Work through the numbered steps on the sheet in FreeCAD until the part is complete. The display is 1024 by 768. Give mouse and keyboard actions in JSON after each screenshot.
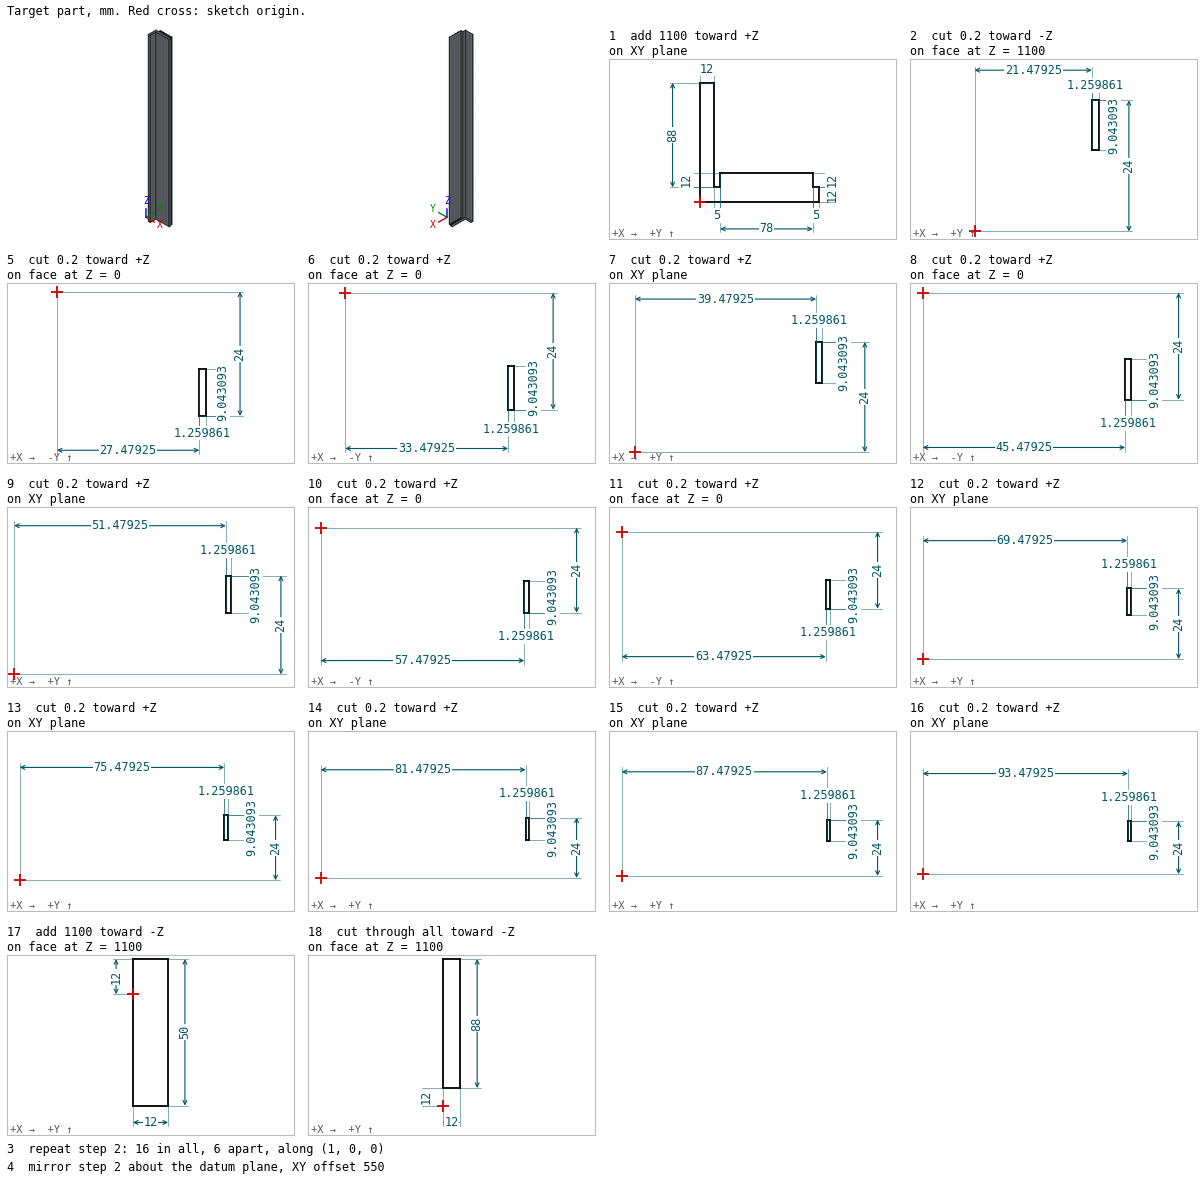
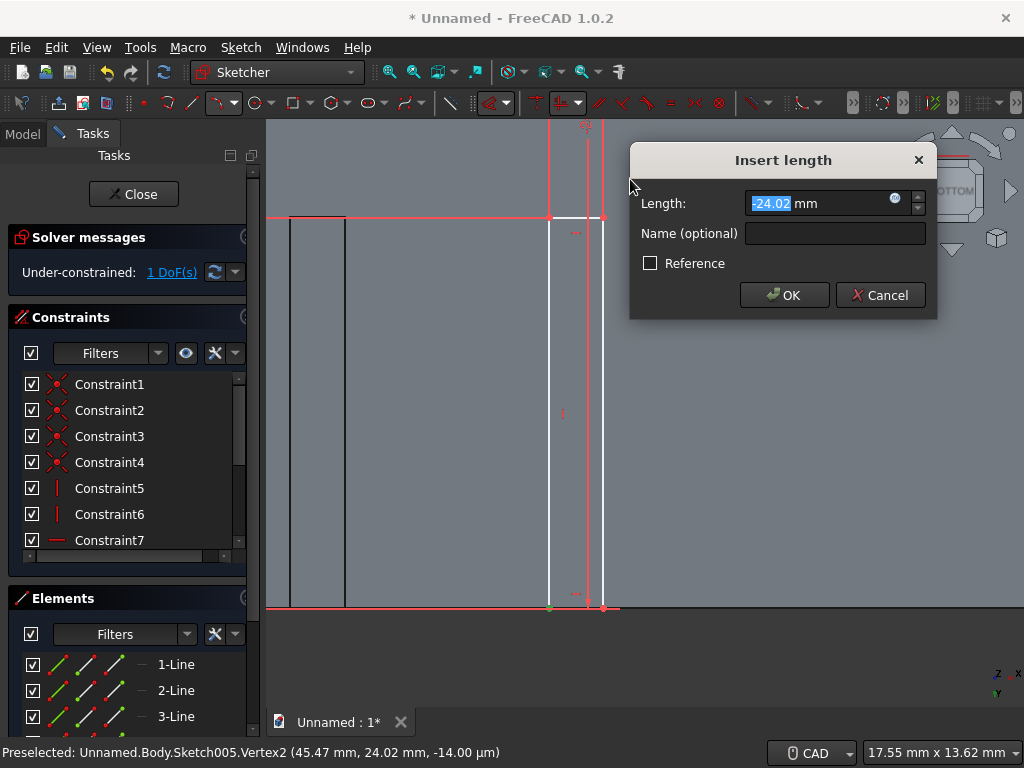
{"action": "type", "text": "-24"}
{"action": "key", "text": "Return"}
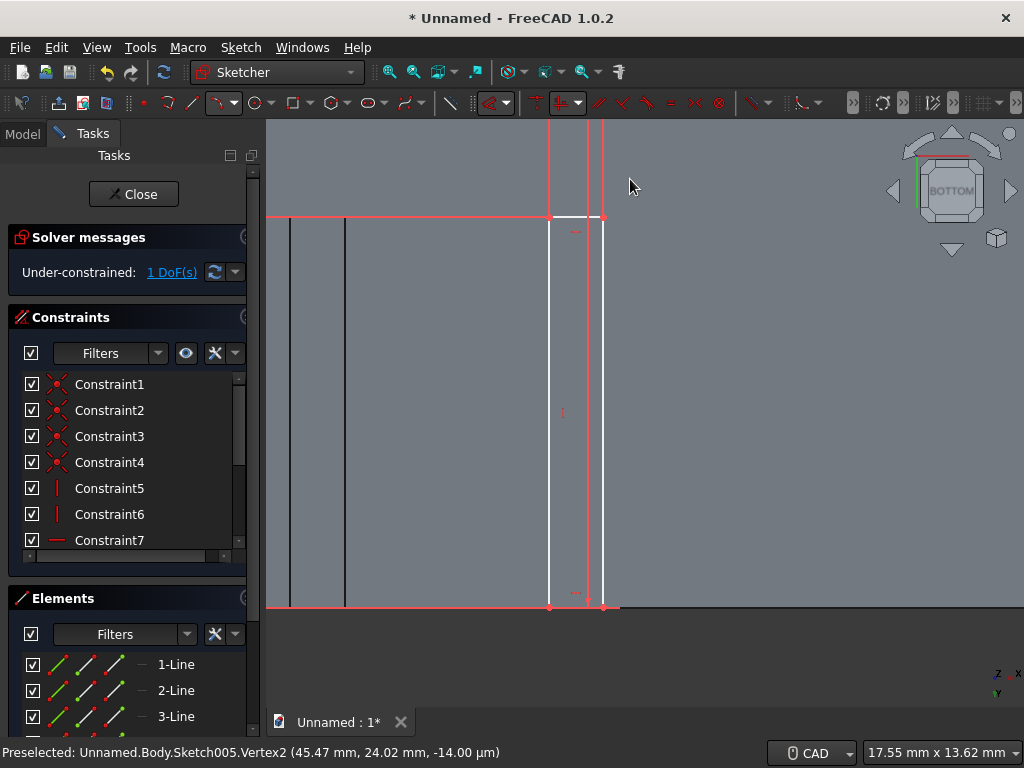
{"action": "left_click", "coordinate": [549, 217]}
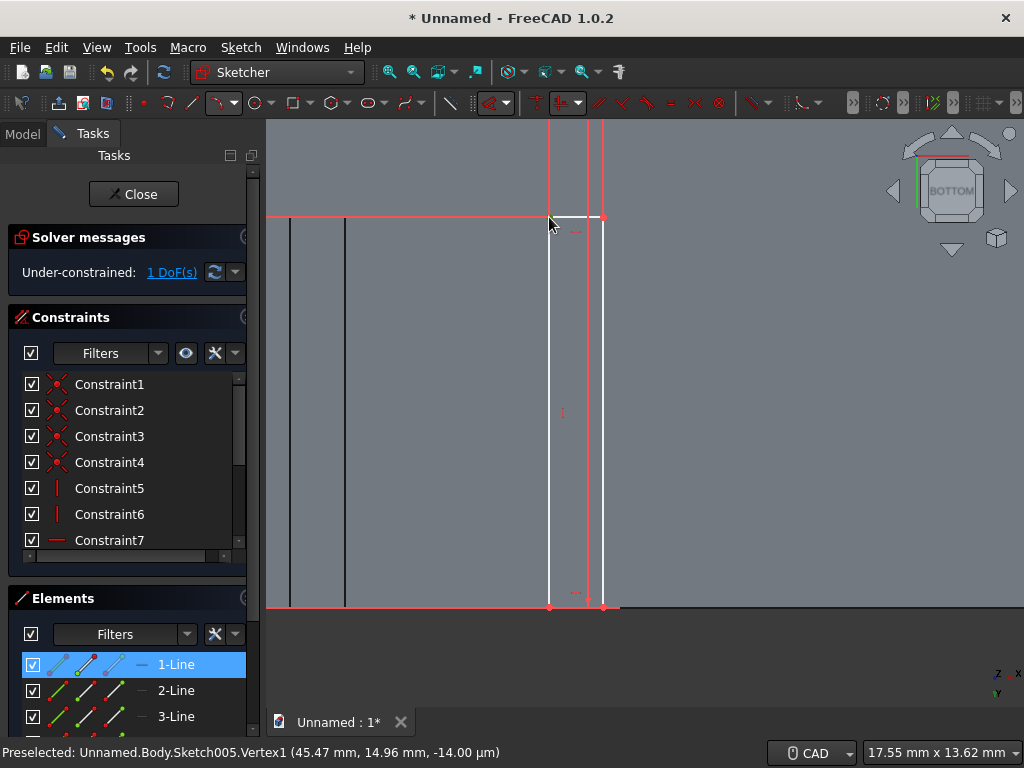
{"action": "left_click", "coordinate": [508, 104]}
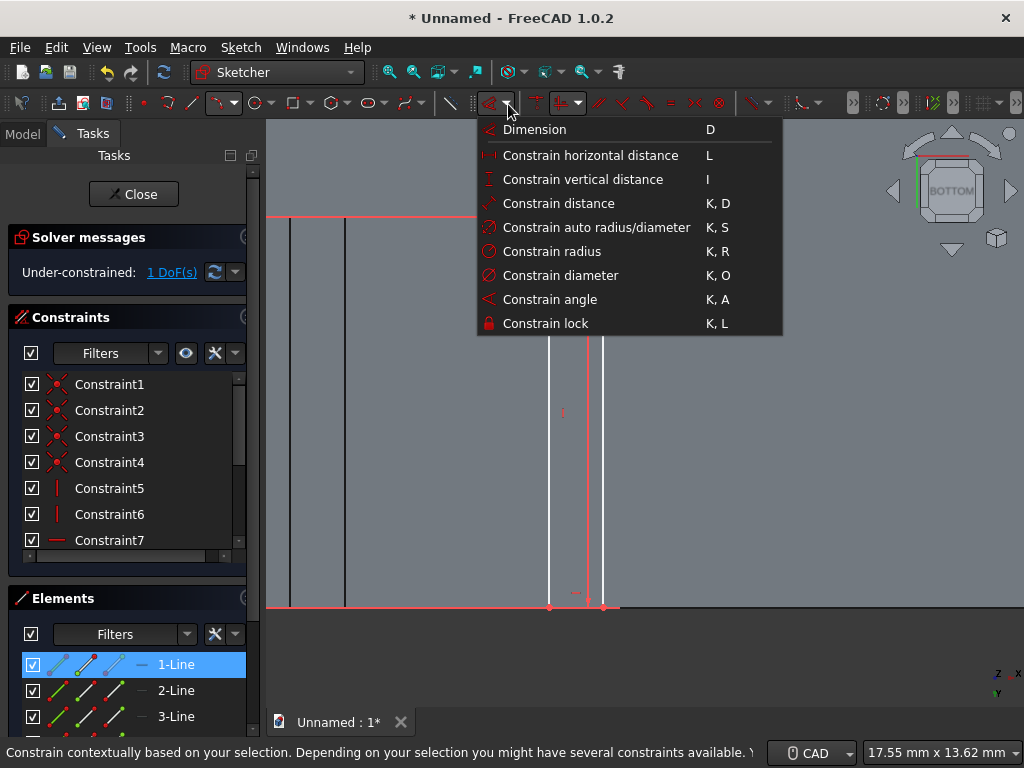
{"action": "left_click", "coordinate": [630, 155]}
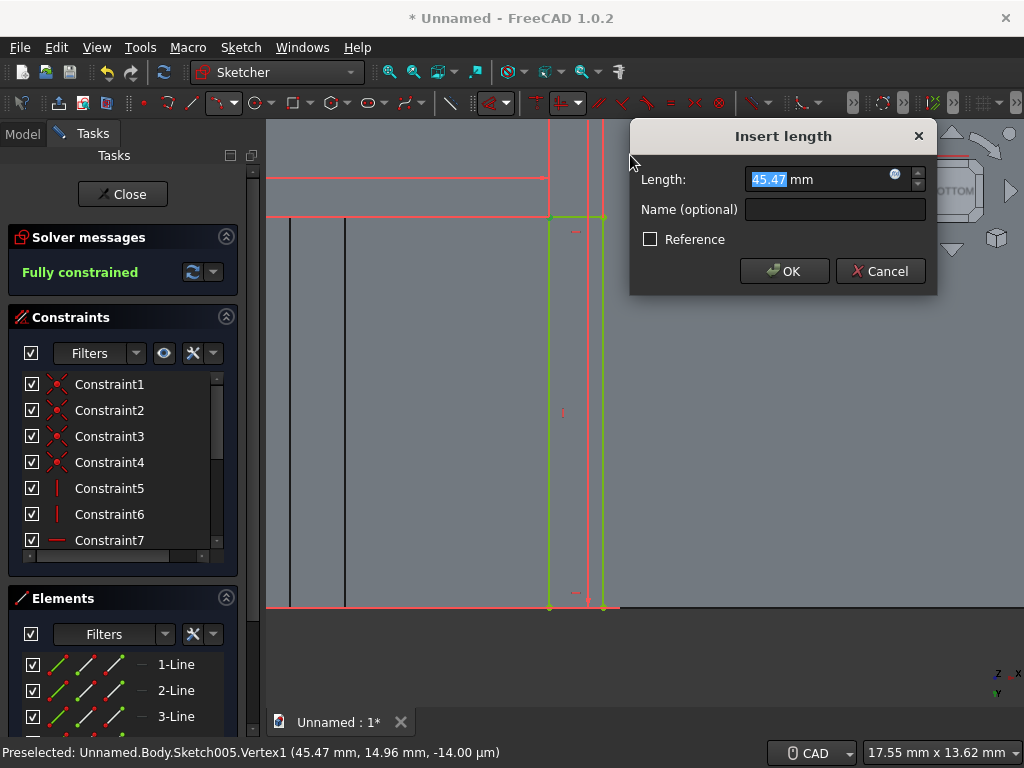
{"action": "type", "text": "45.47925"}
{"action": "key", "text": "Return"}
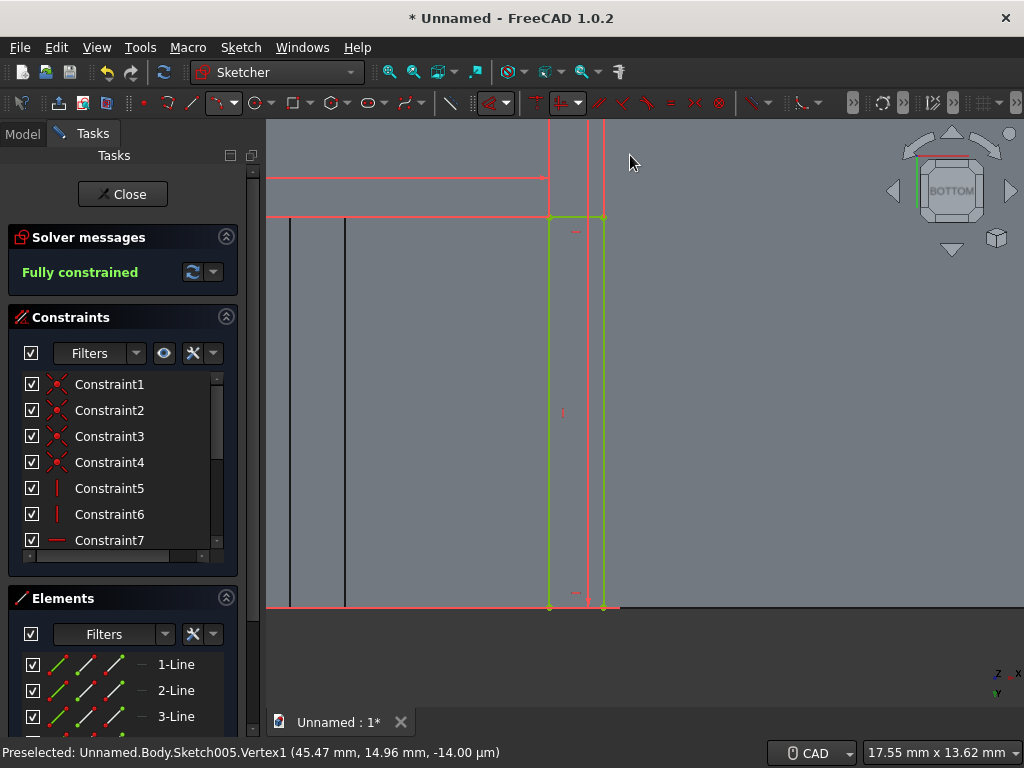
{"action": "left_click", "coordinate": [123, 194]}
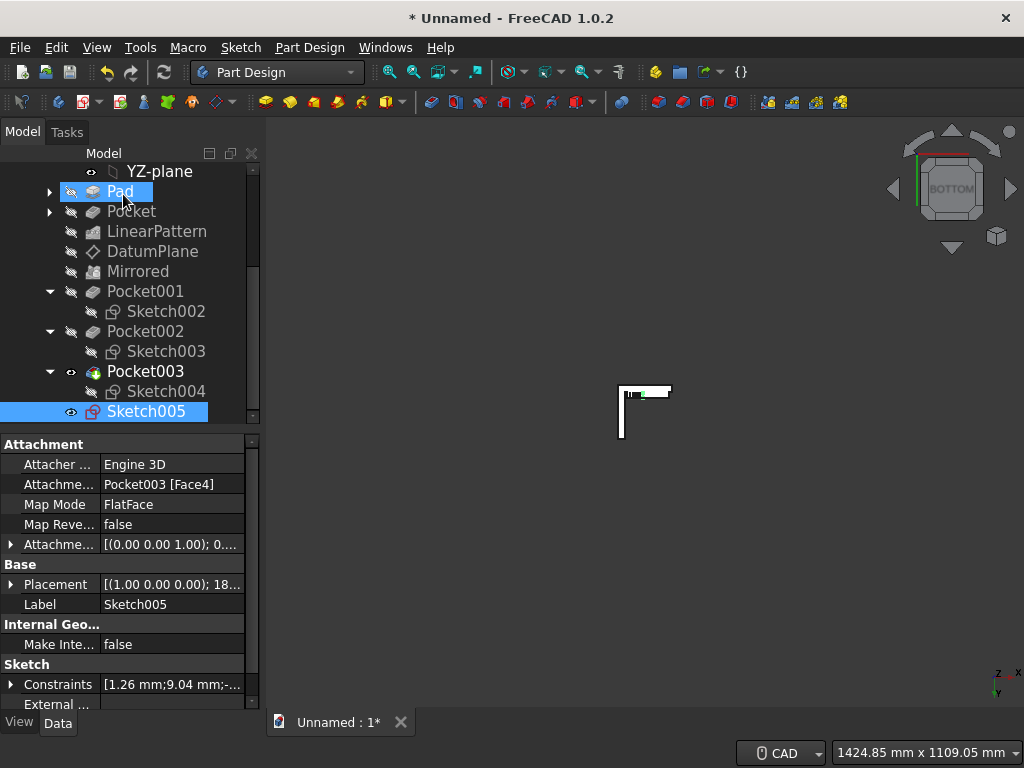
{"action": "left_click", "coordinate": [432, 102]}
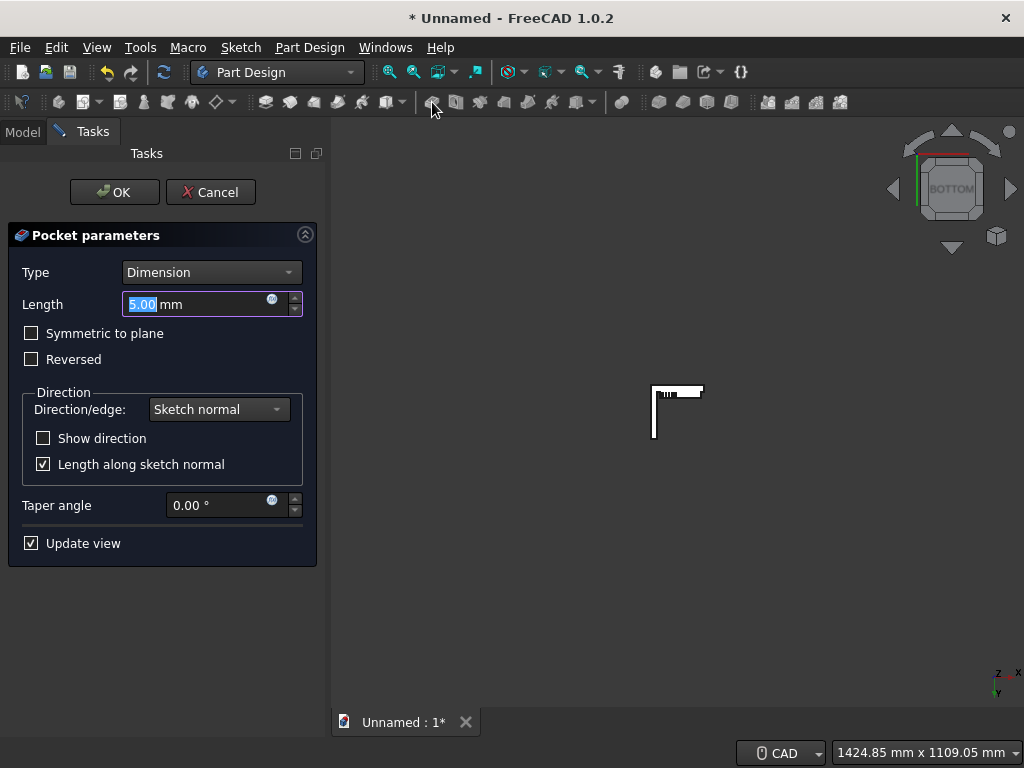
{"action": "type", "text": "0.2"}
{"action": "key", "text": "Tab"}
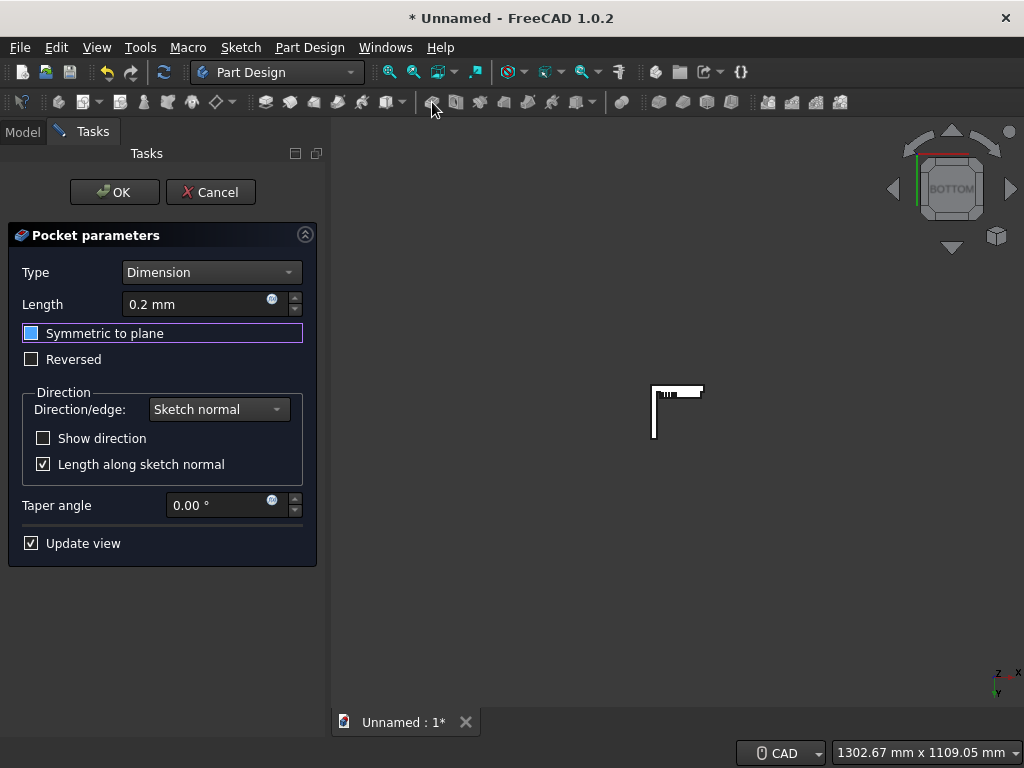
{"action": "left_click", "coordinate": [115, 192]}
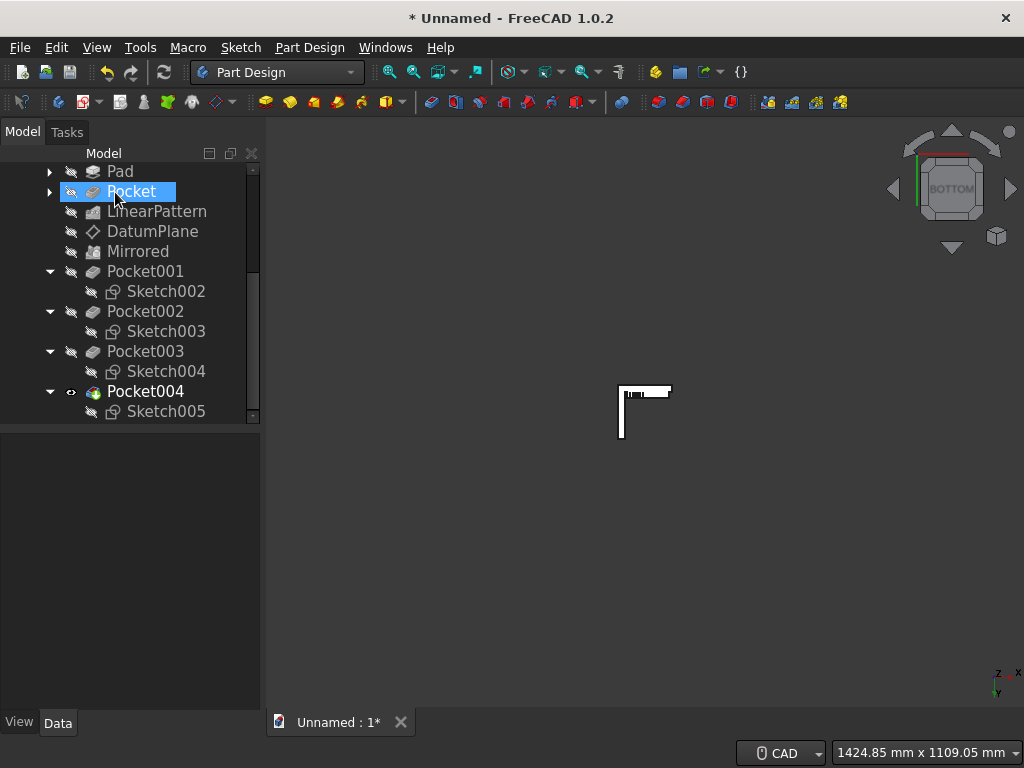
{"action": "left_click", "coordinate": [390, 72]}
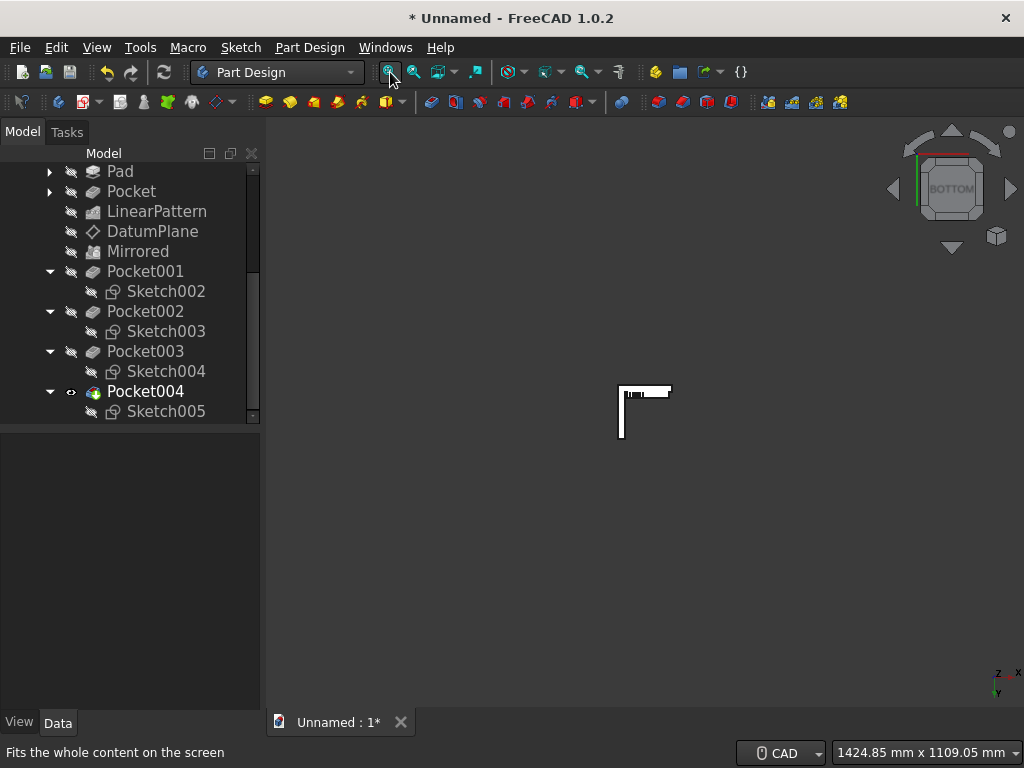
{"action": "left_click", "coordinate": [84, 102]}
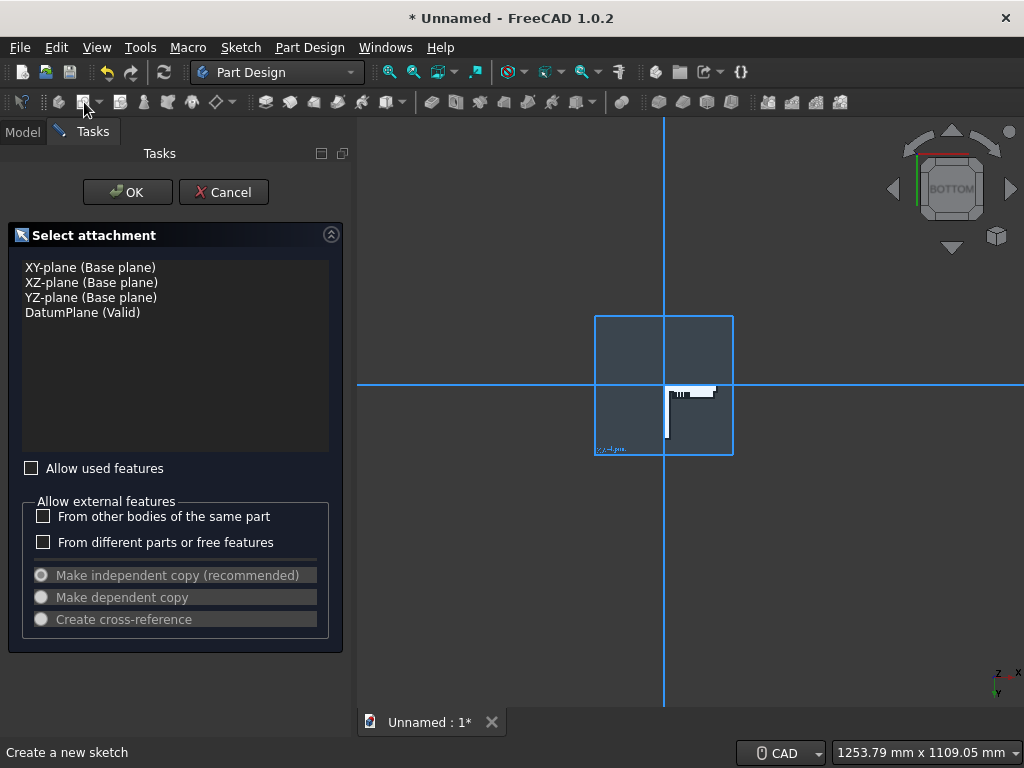
{"action": "left_click", "coordinate": [82, 268]}